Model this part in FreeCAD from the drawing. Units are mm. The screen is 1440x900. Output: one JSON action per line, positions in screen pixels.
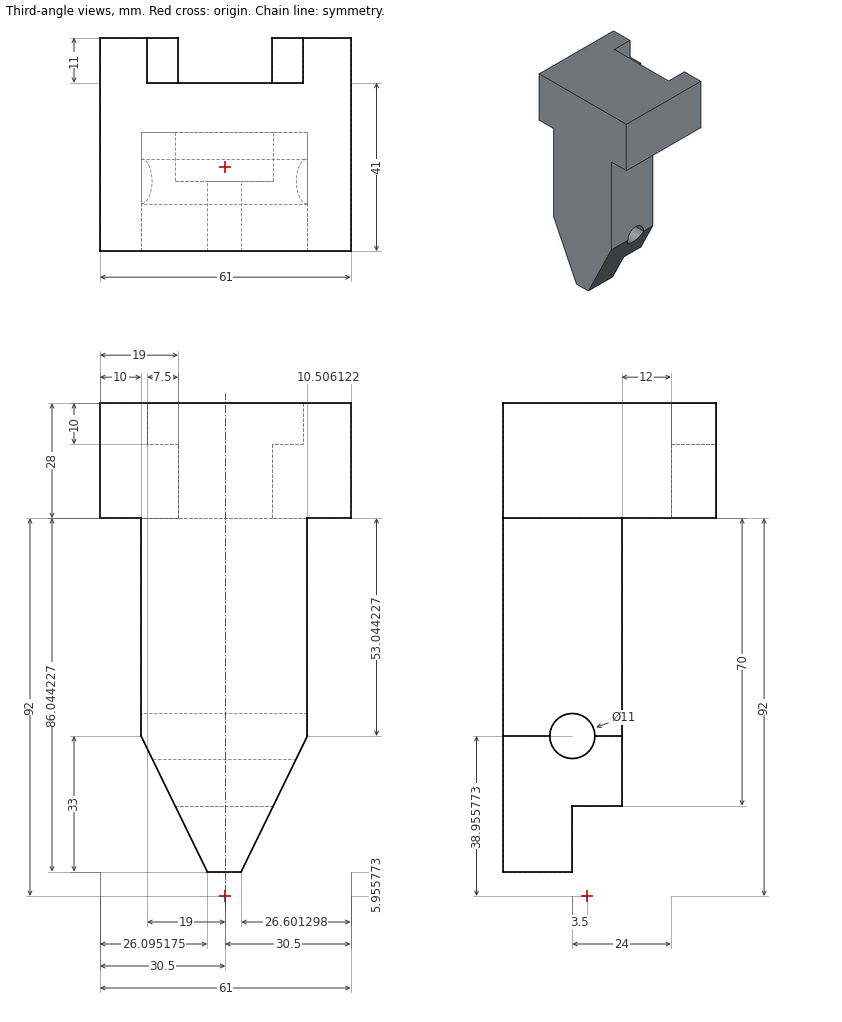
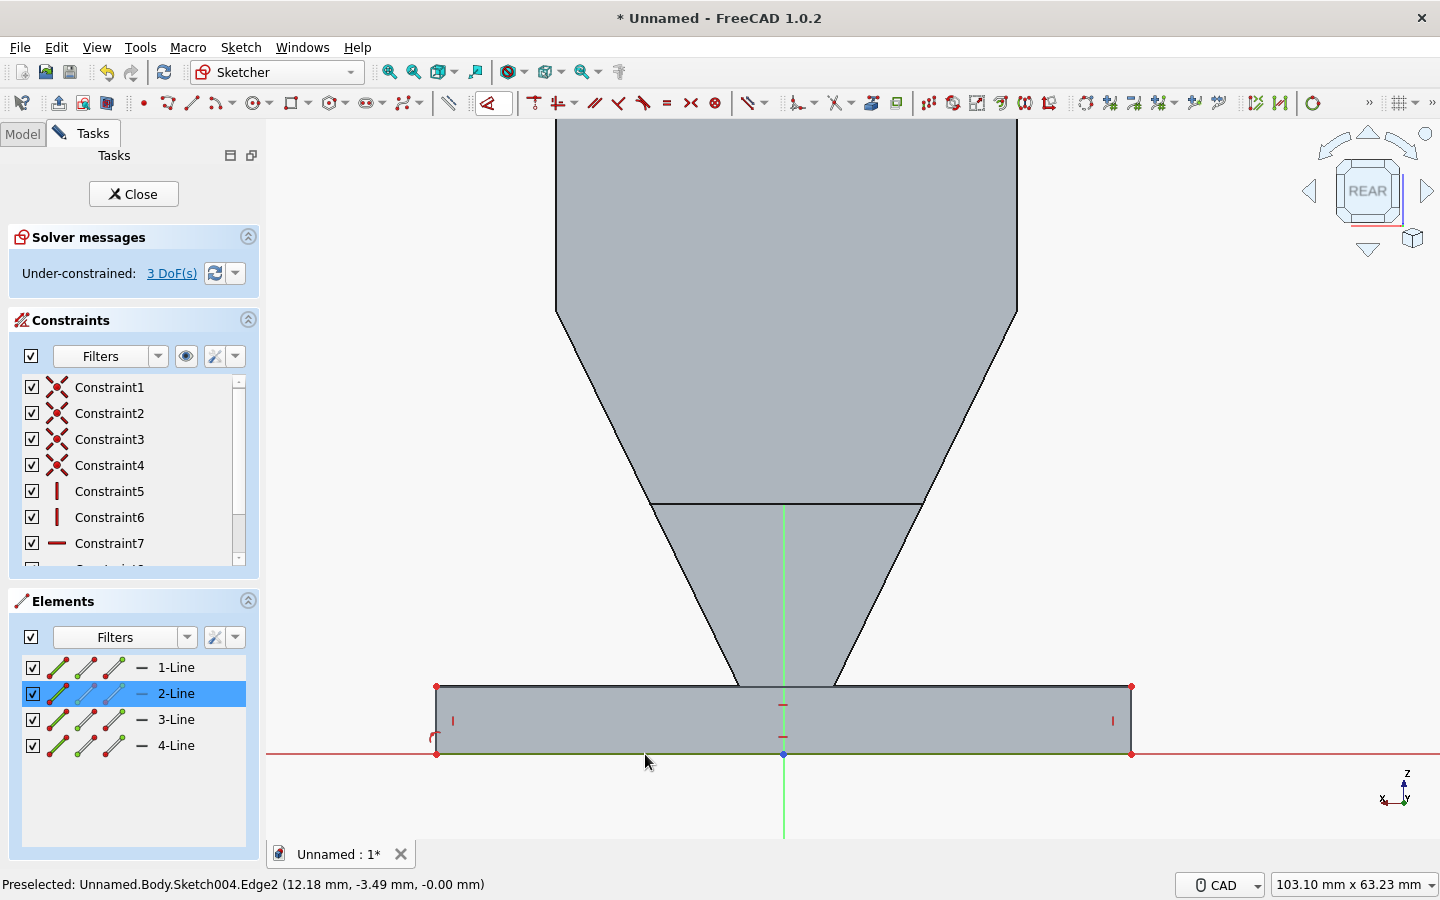
{"action": "left_click", "coordinate": [506, 104]}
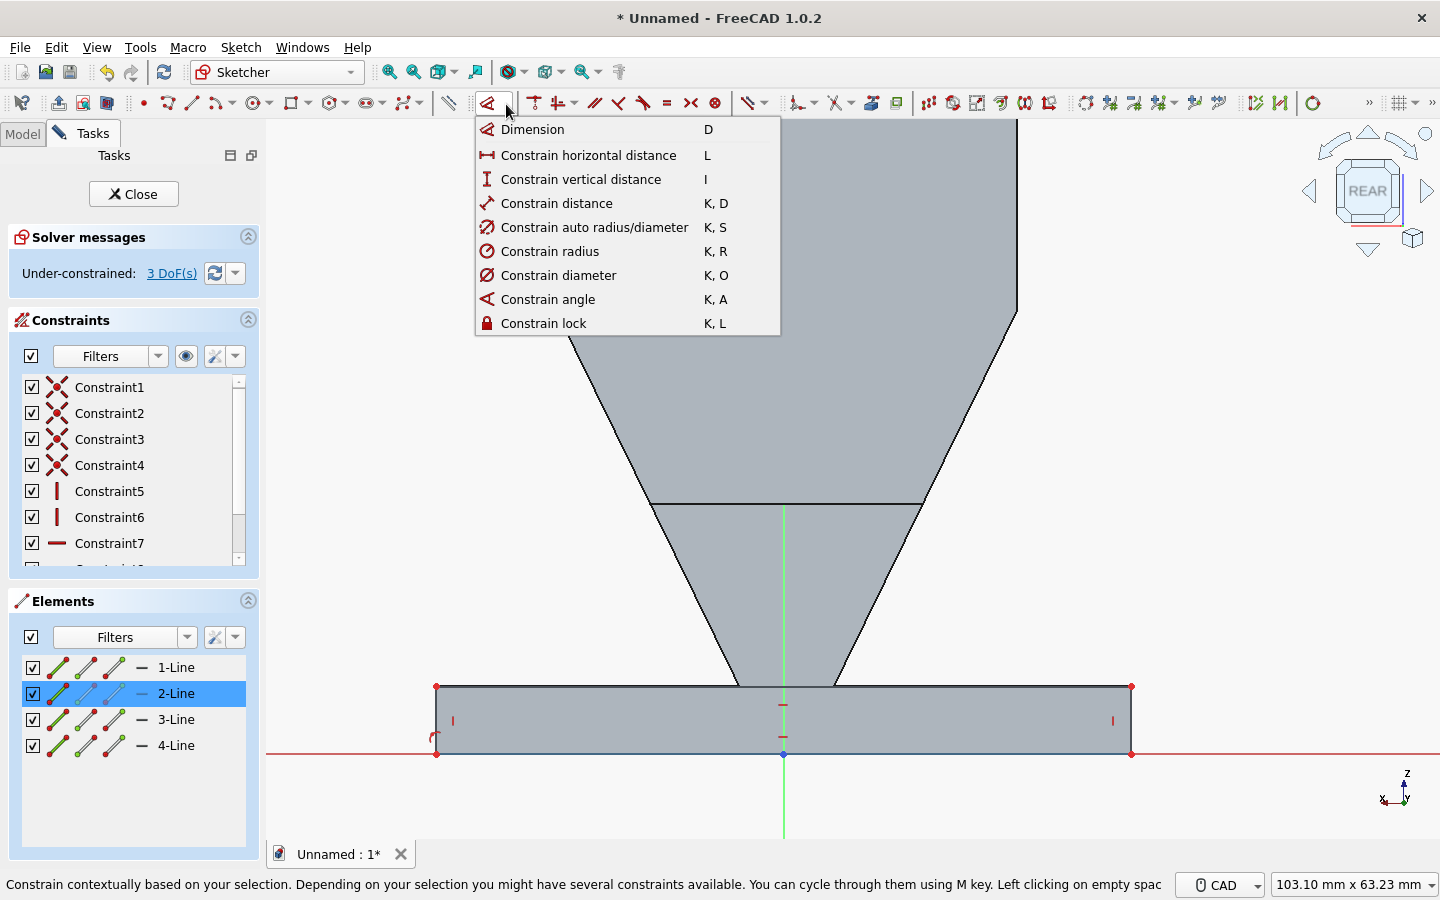
{"action": "left_click", "coordinate": [628, 155]}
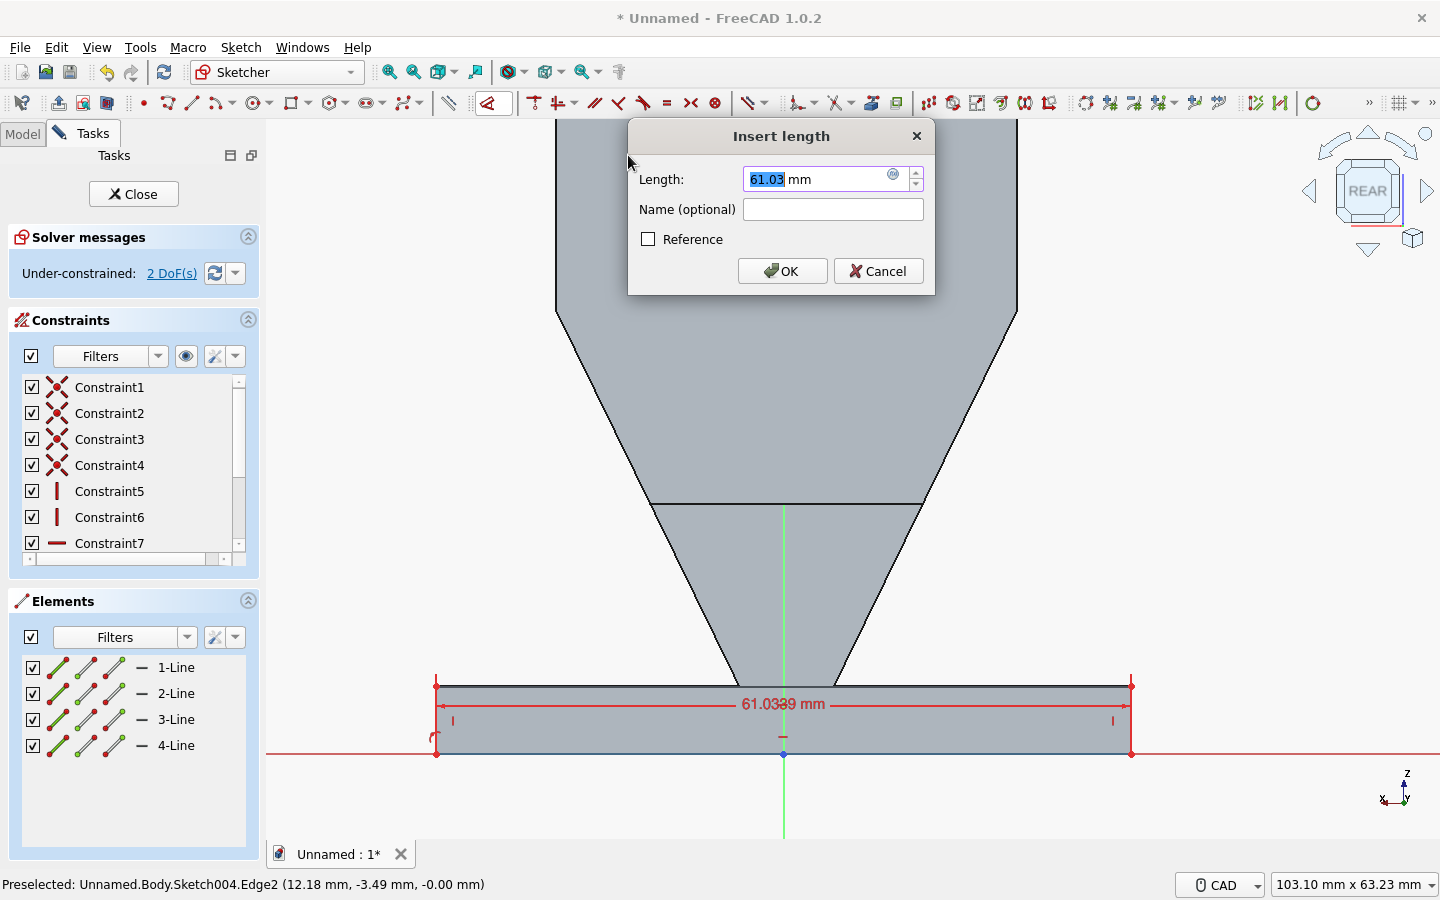
{"action": "type", "text": "61"}
{"action": "key", "text": "Return"}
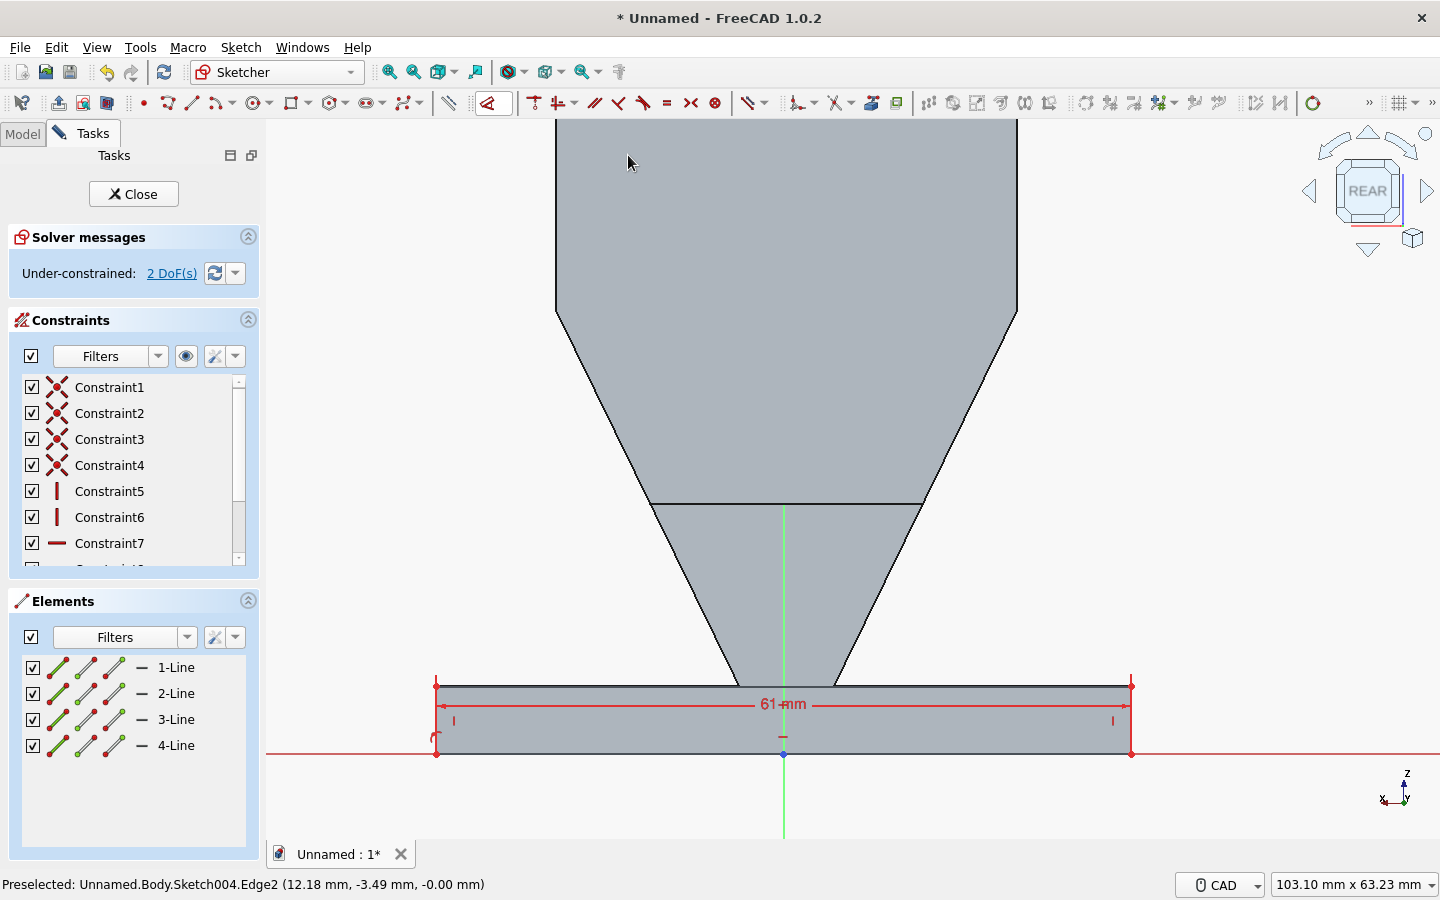
{"action": "left_click", "coordinate": [436, 687]}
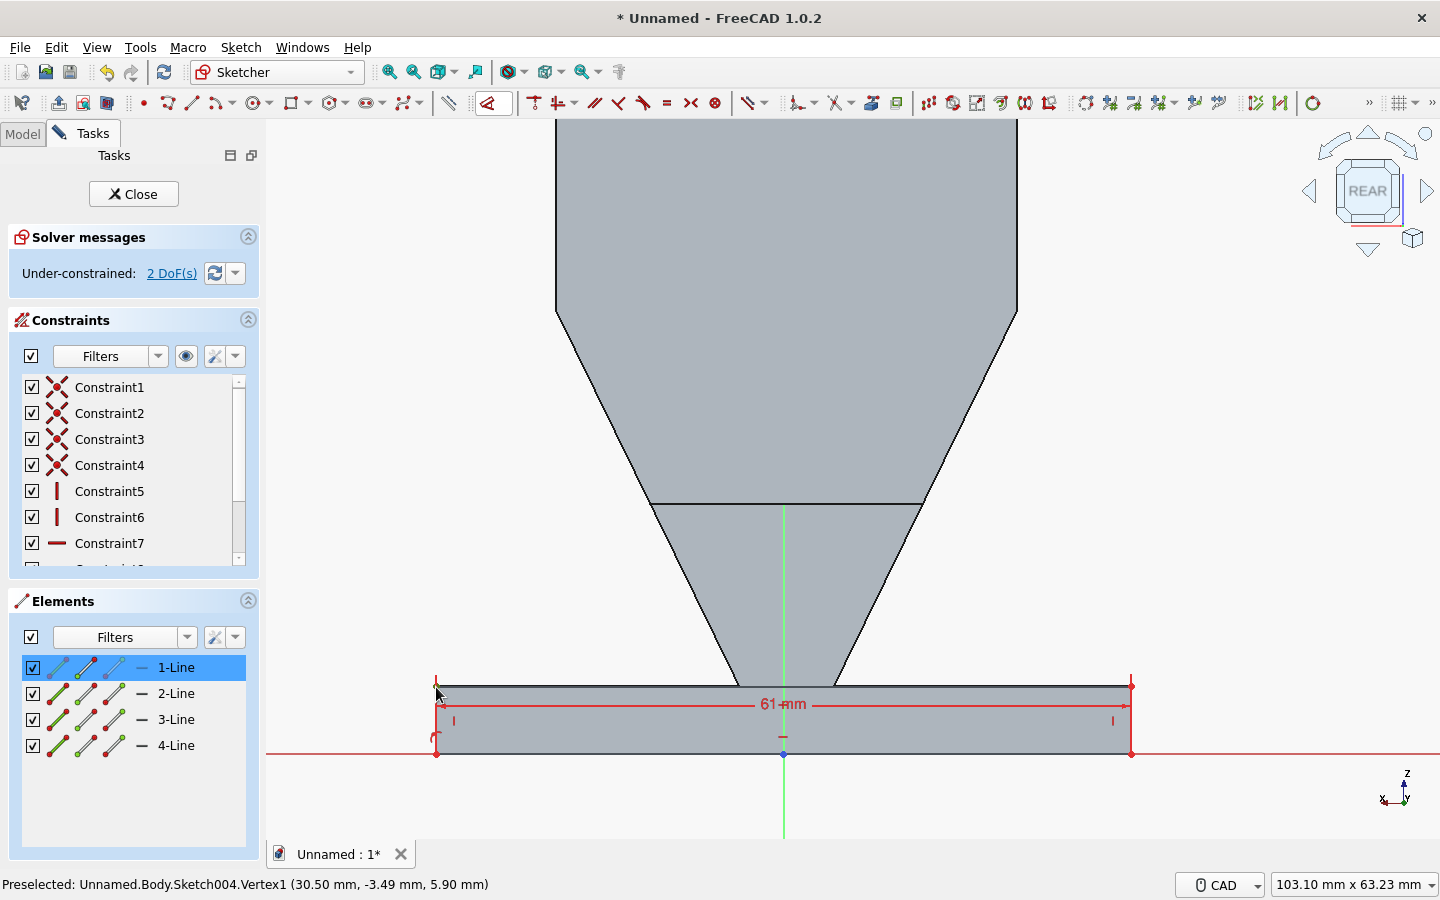
{"action": "left_click", "coordinate": [506, 104]}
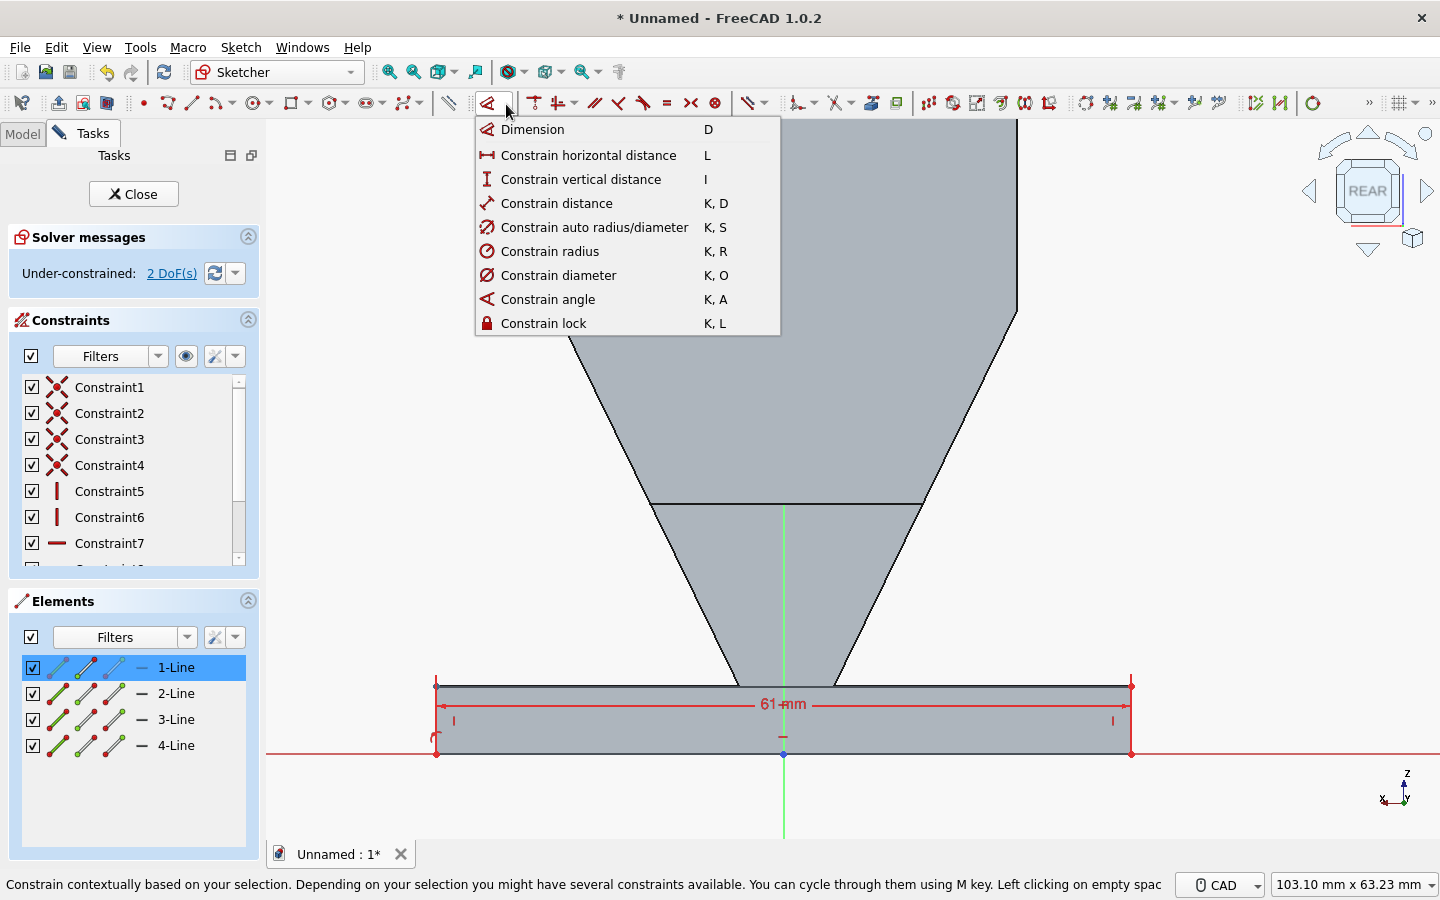
{"action": "left_click", "coordinate": [628, 155]}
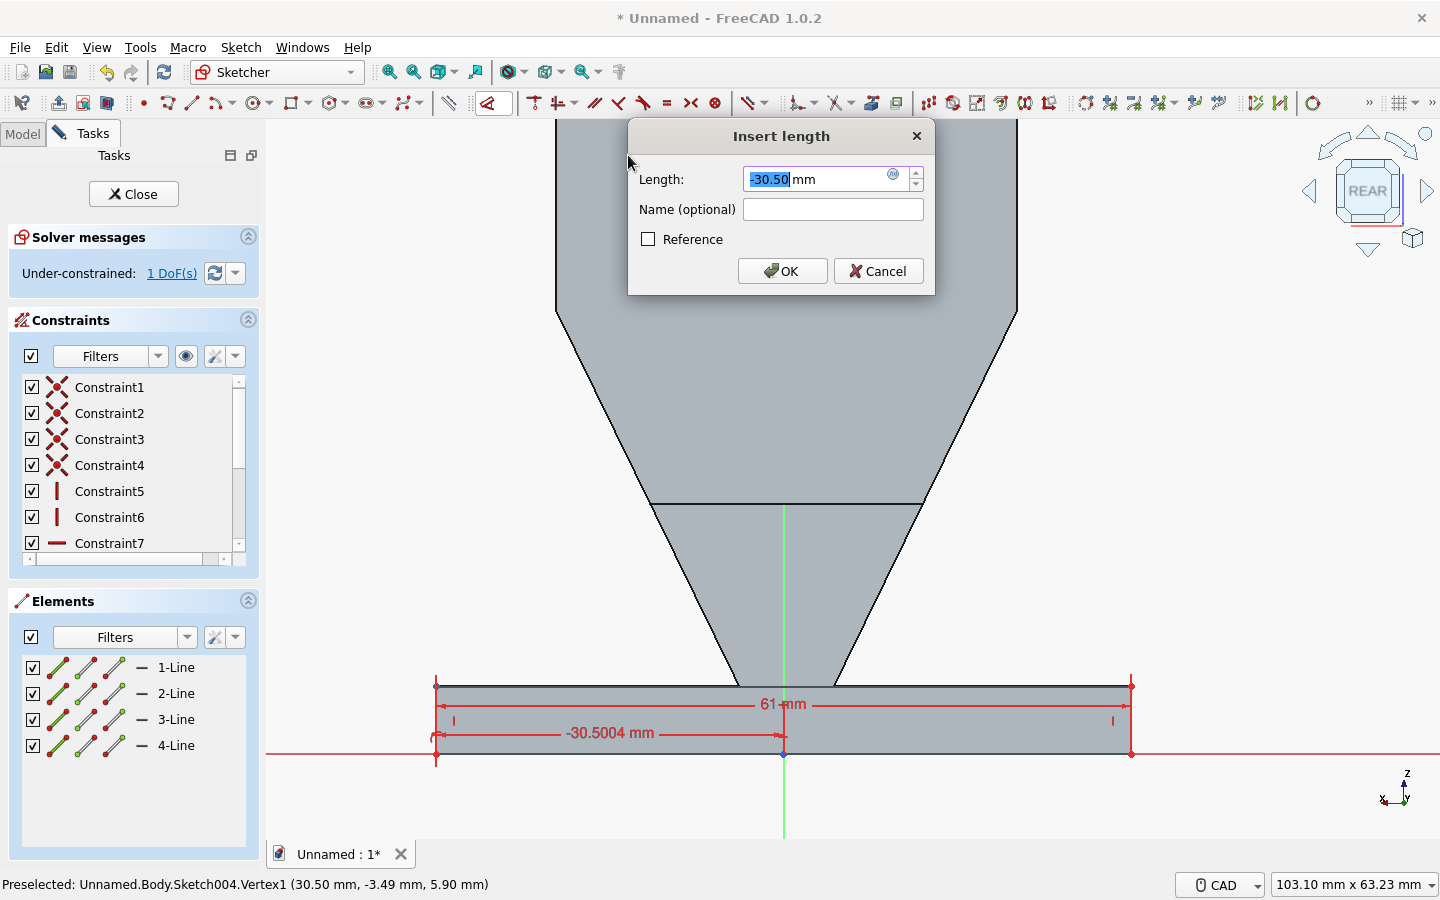
{"action": "type", "text": "-30.5"}
{"action": "key", "text": "Return"}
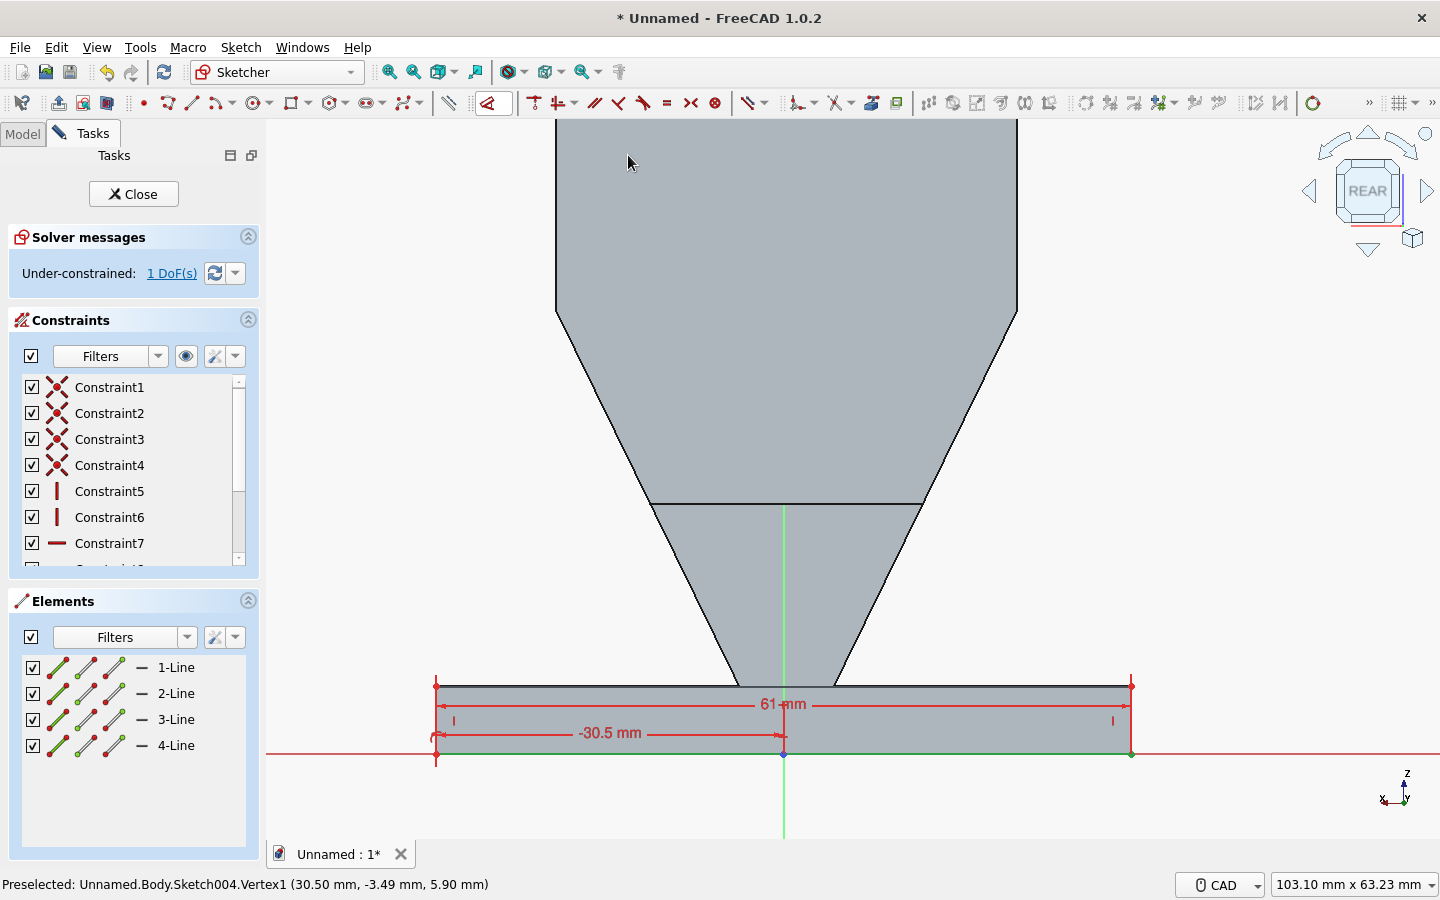
{"action": "left_click", "coordinate": [436, 707]}